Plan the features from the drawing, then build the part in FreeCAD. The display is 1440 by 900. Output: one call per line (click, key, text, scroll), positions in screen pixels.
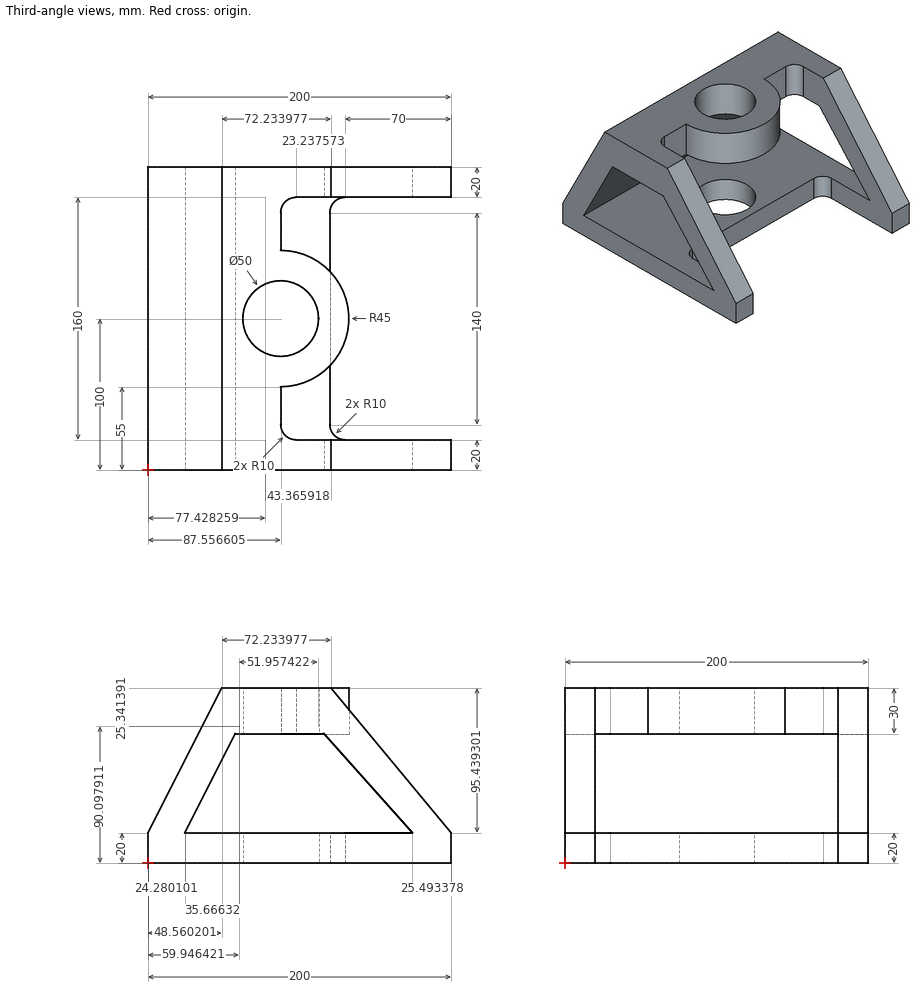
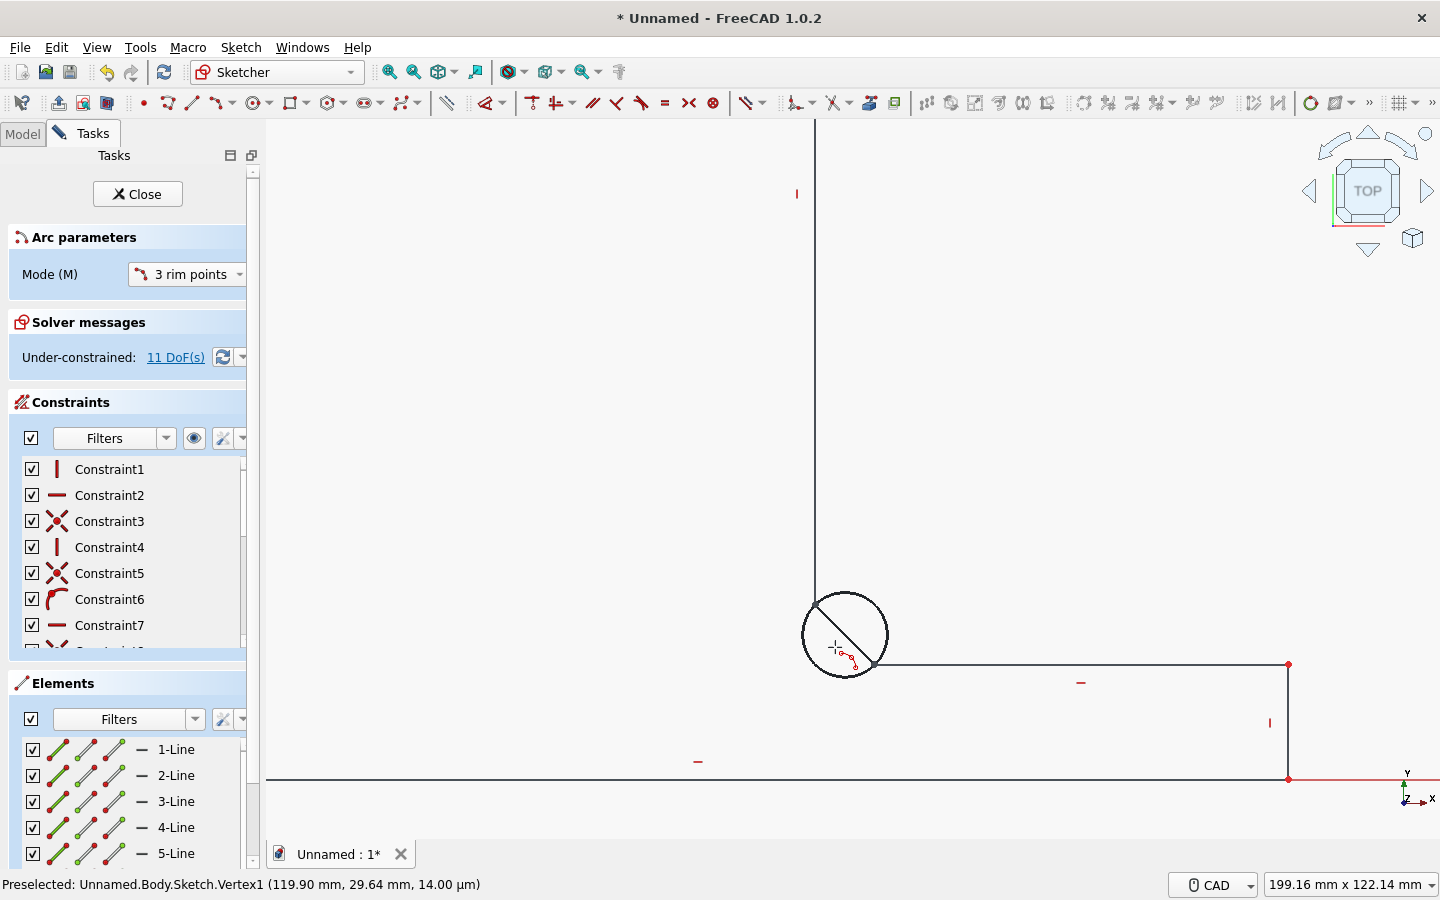
click(833, 645)
key(Escape)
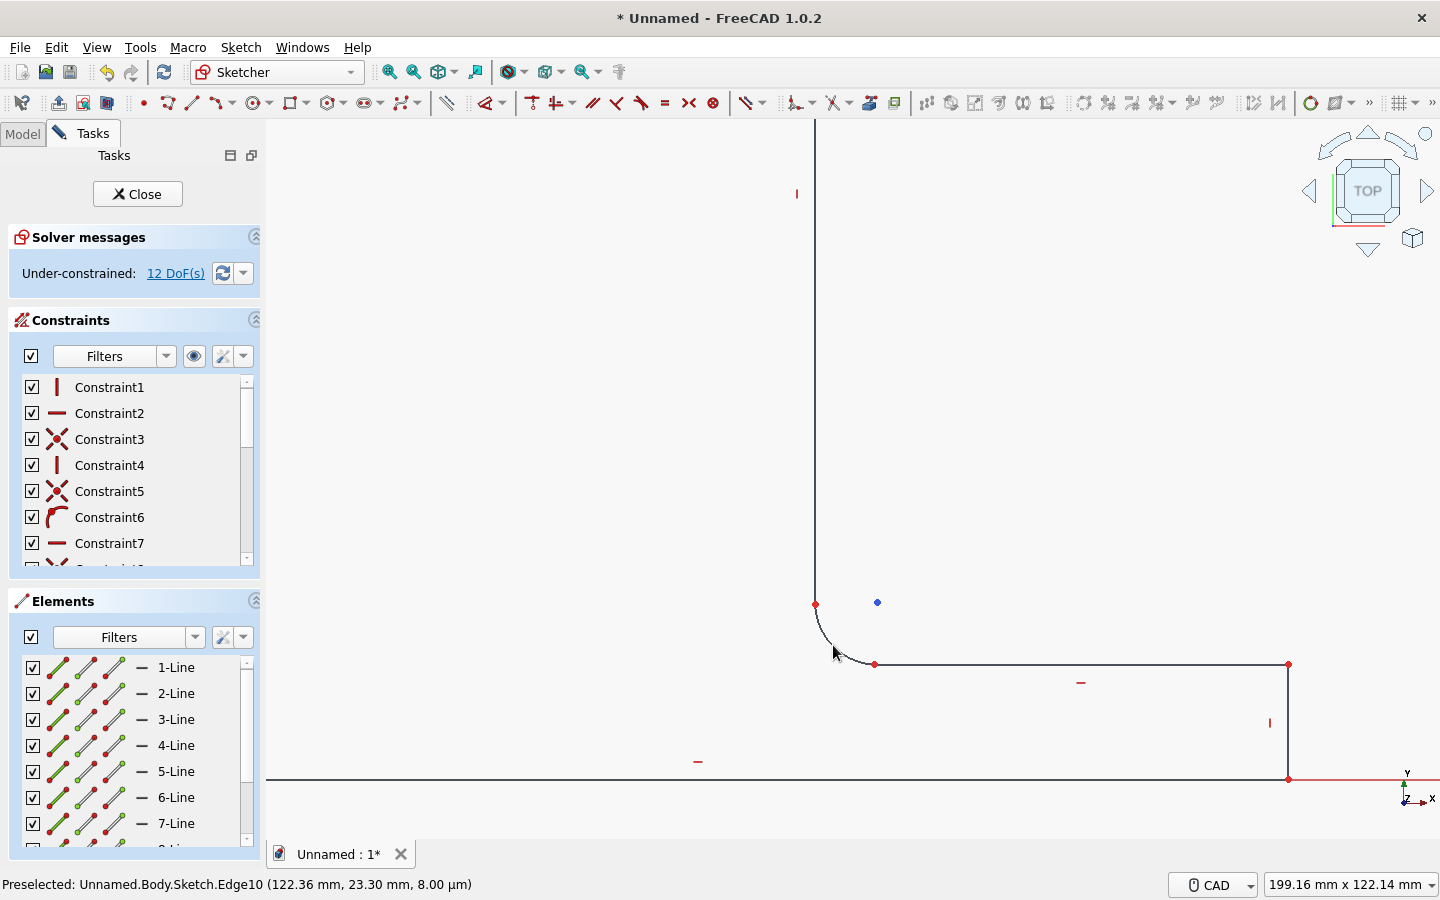
click(815, 358)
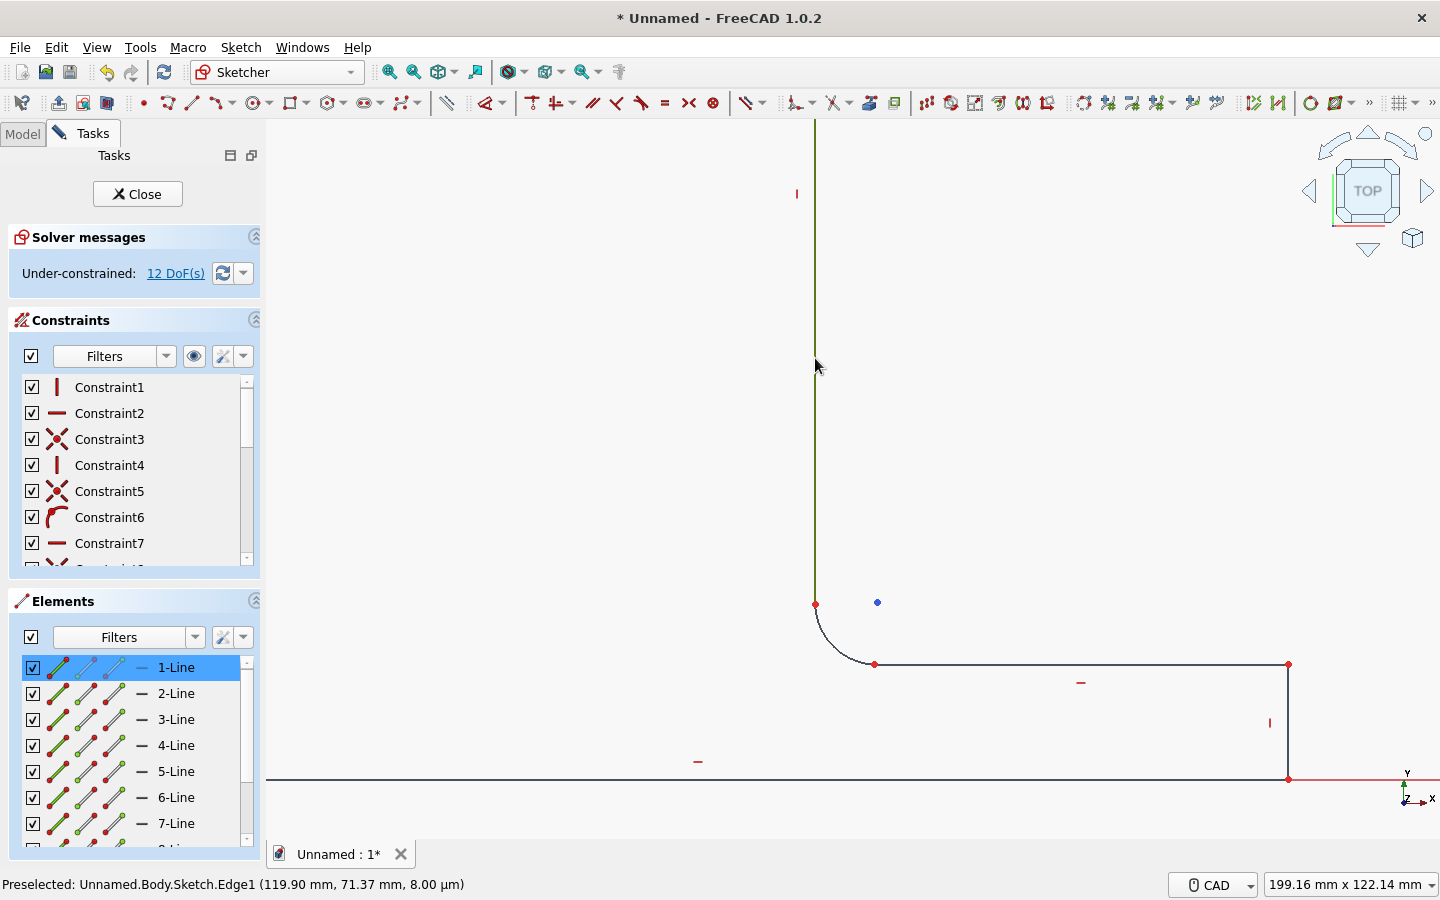
scroll(835, 647, down, 5)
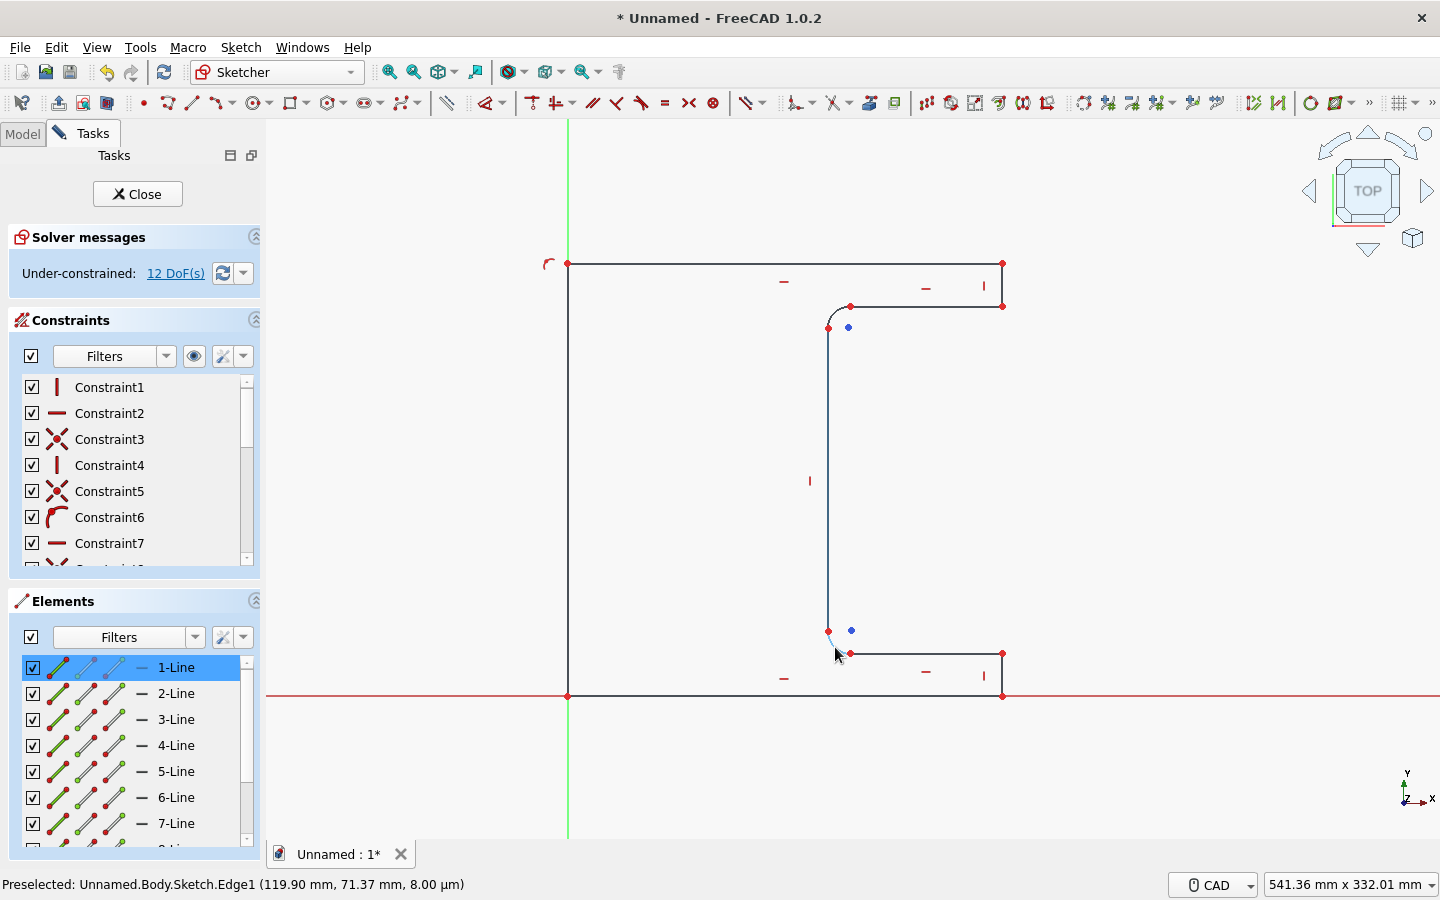
scroll(840, 309, up, 2)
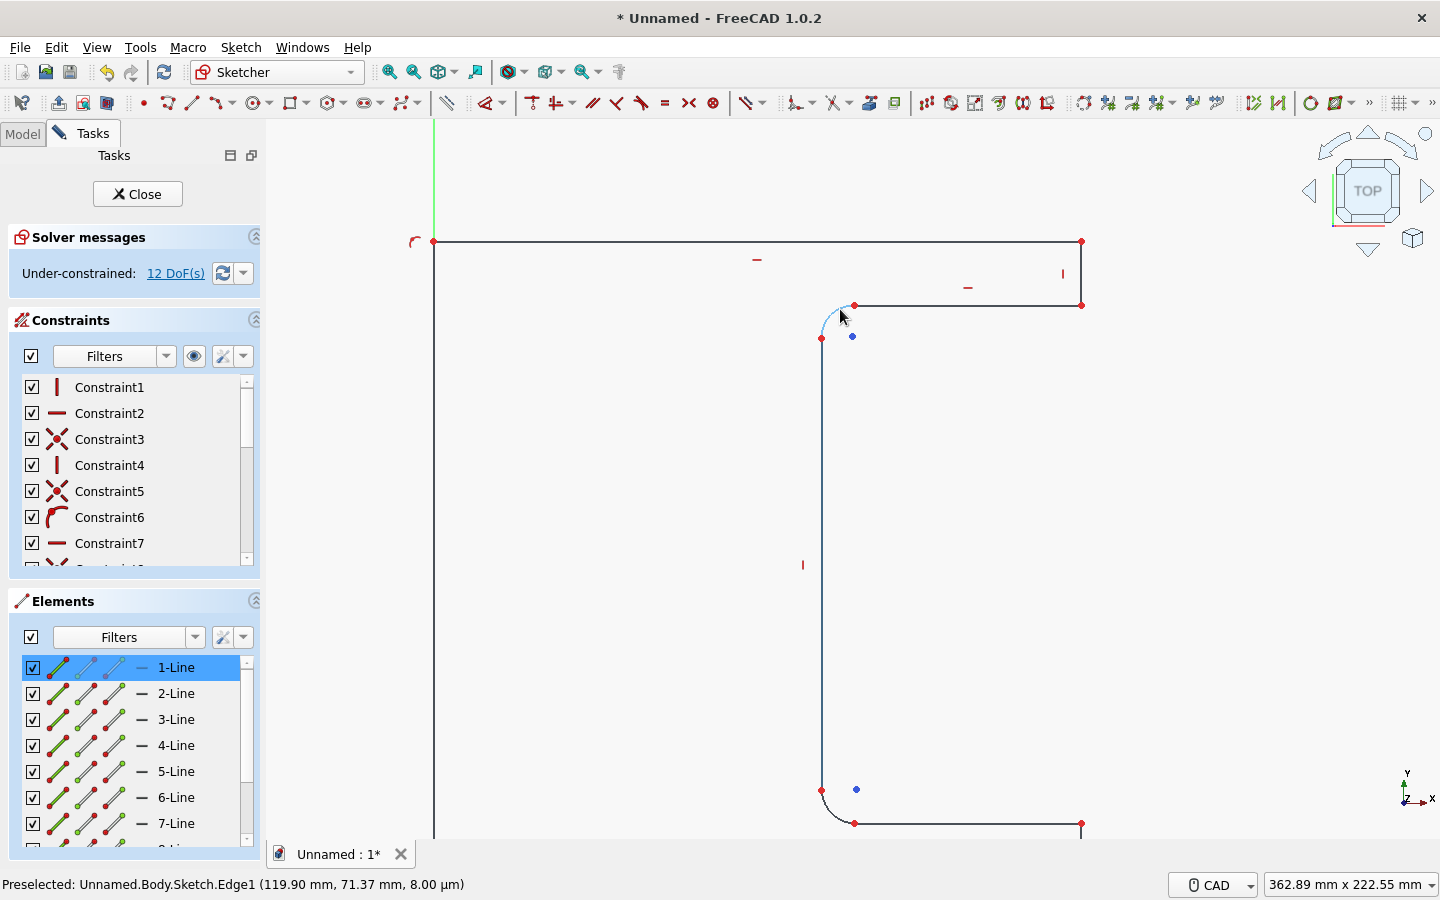
click(839, 309)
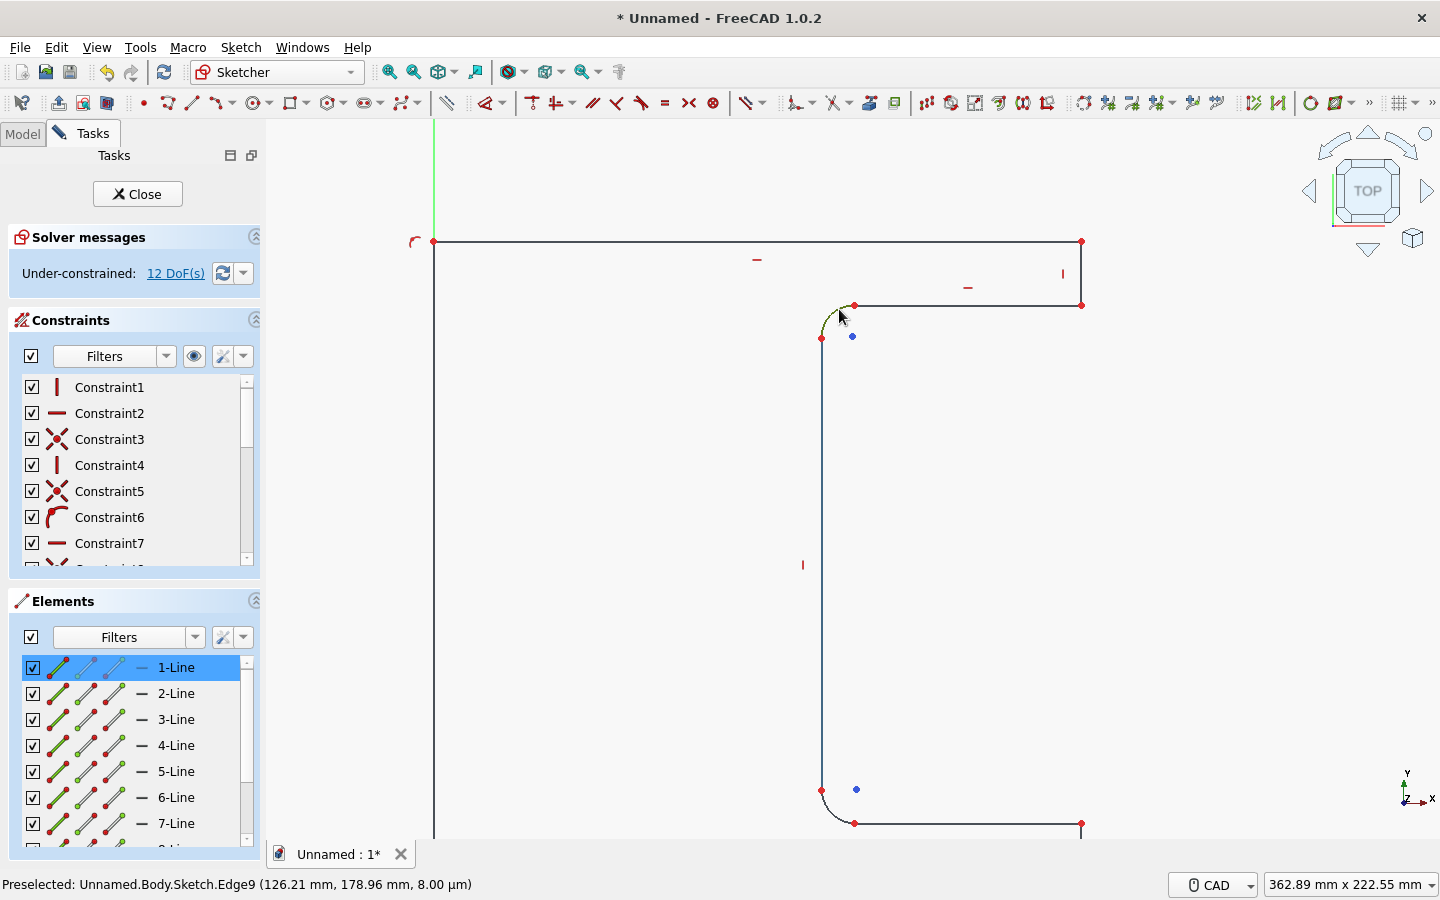
click(642, 104)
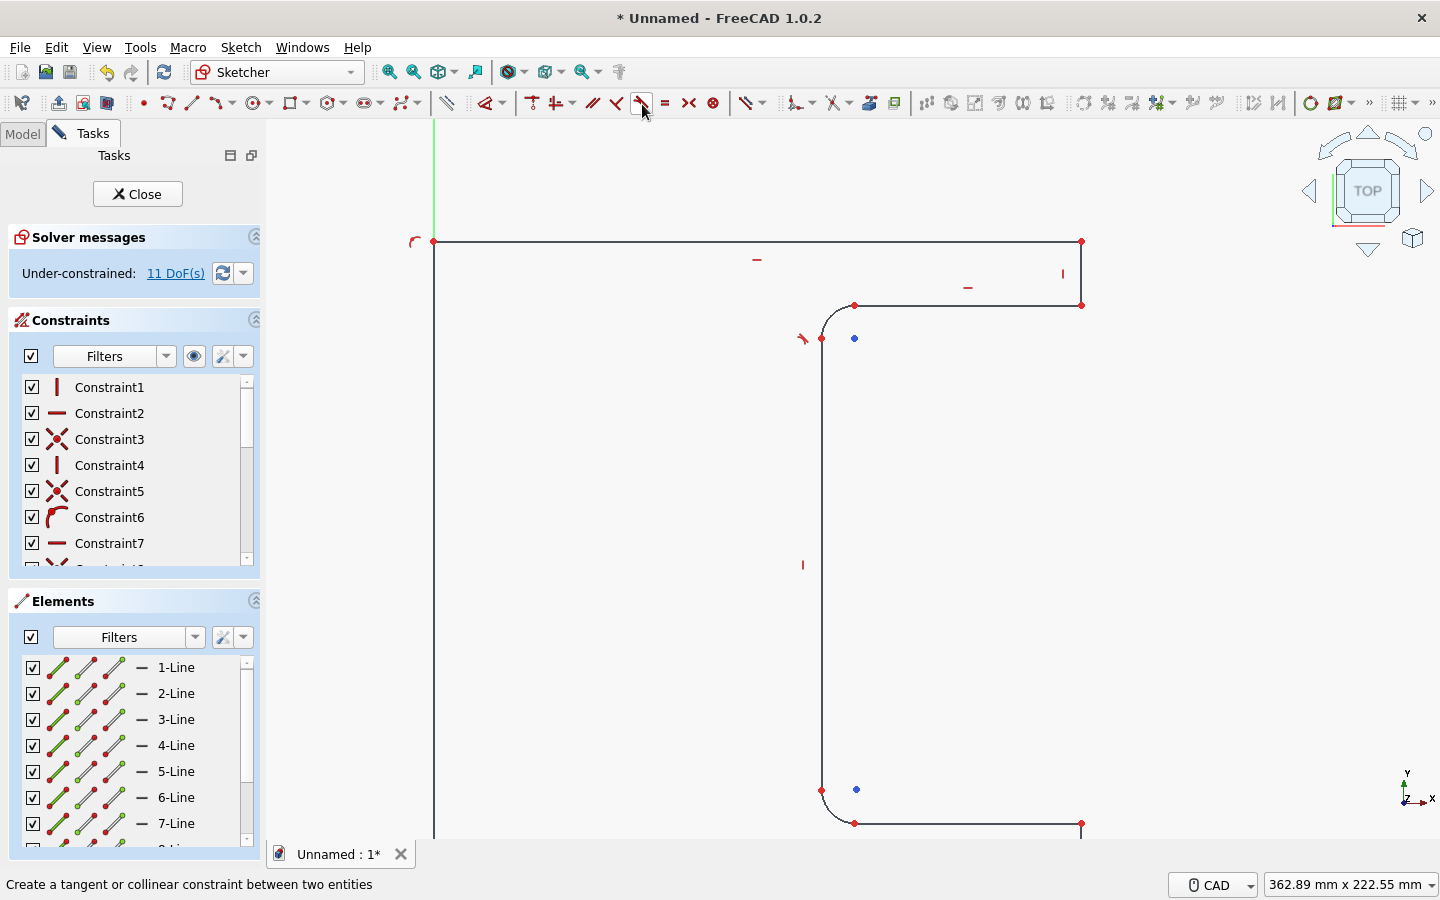
click(822, 655)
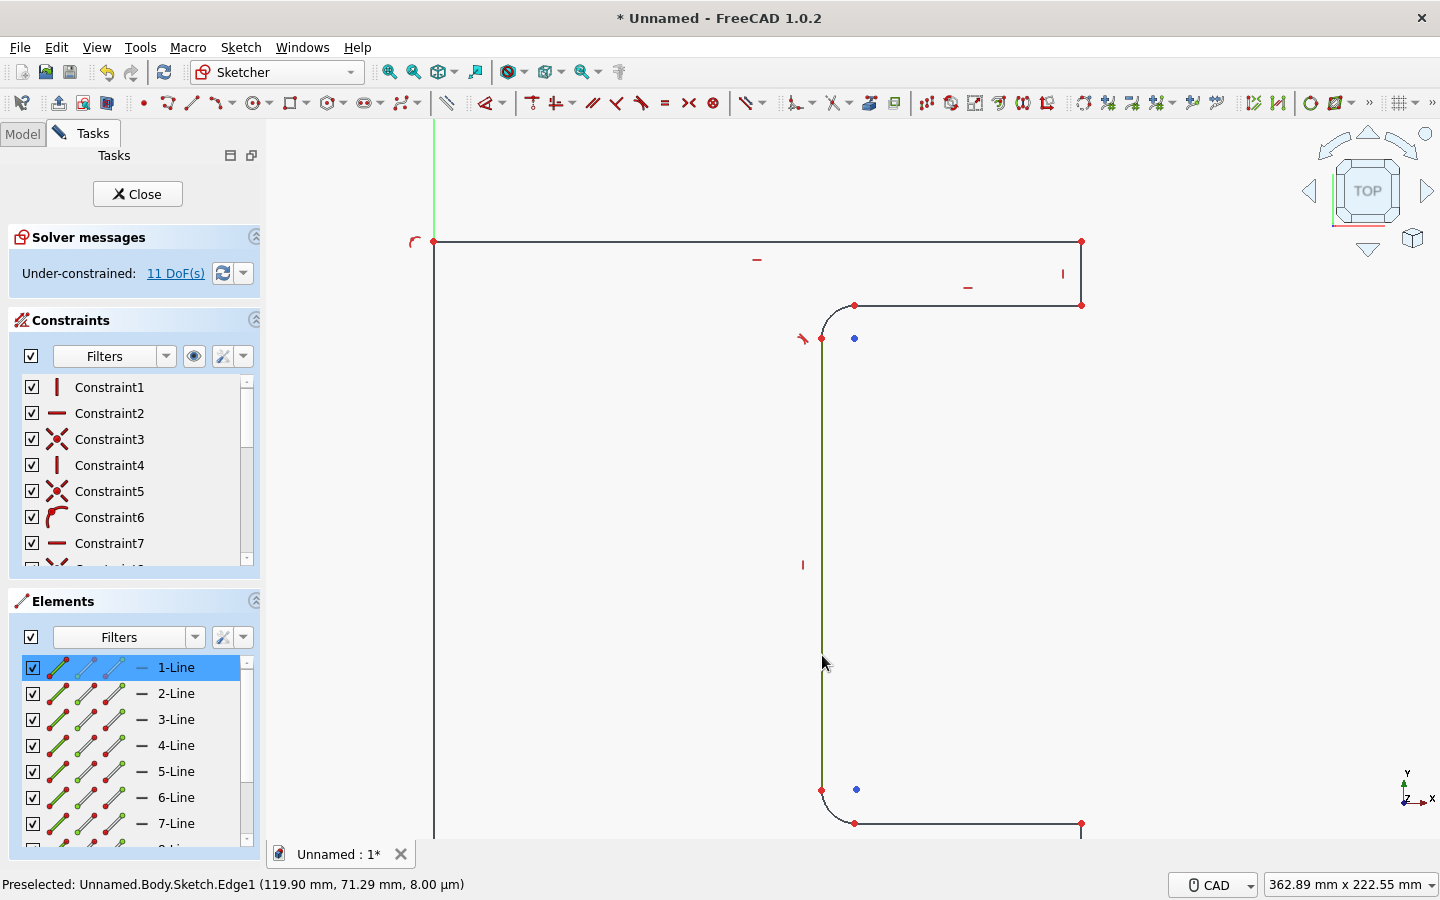
click(826, 805)